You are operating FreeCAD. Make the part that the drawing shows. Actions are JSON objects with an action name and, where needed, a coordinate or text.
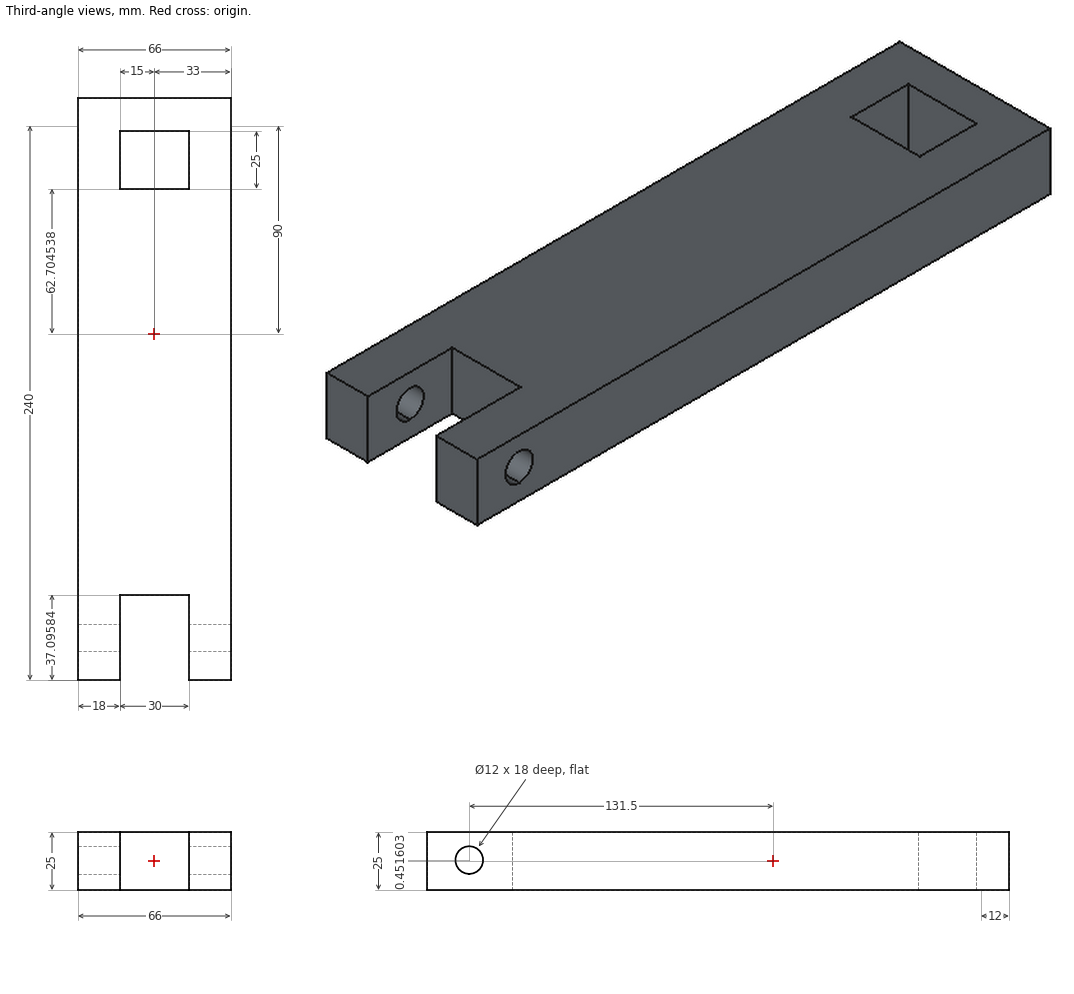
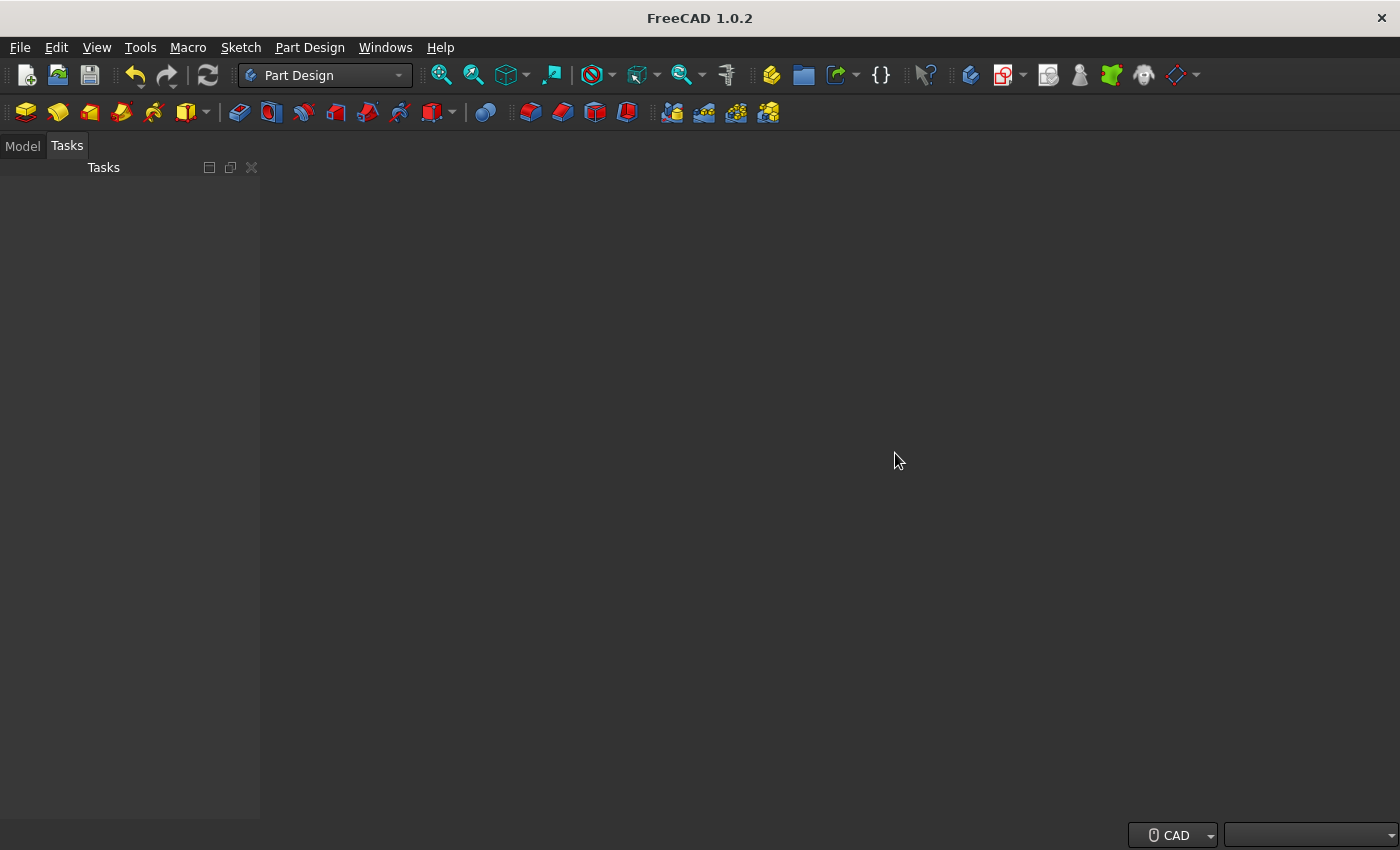
{"action": "left_click", "coordinate": [26, 76]}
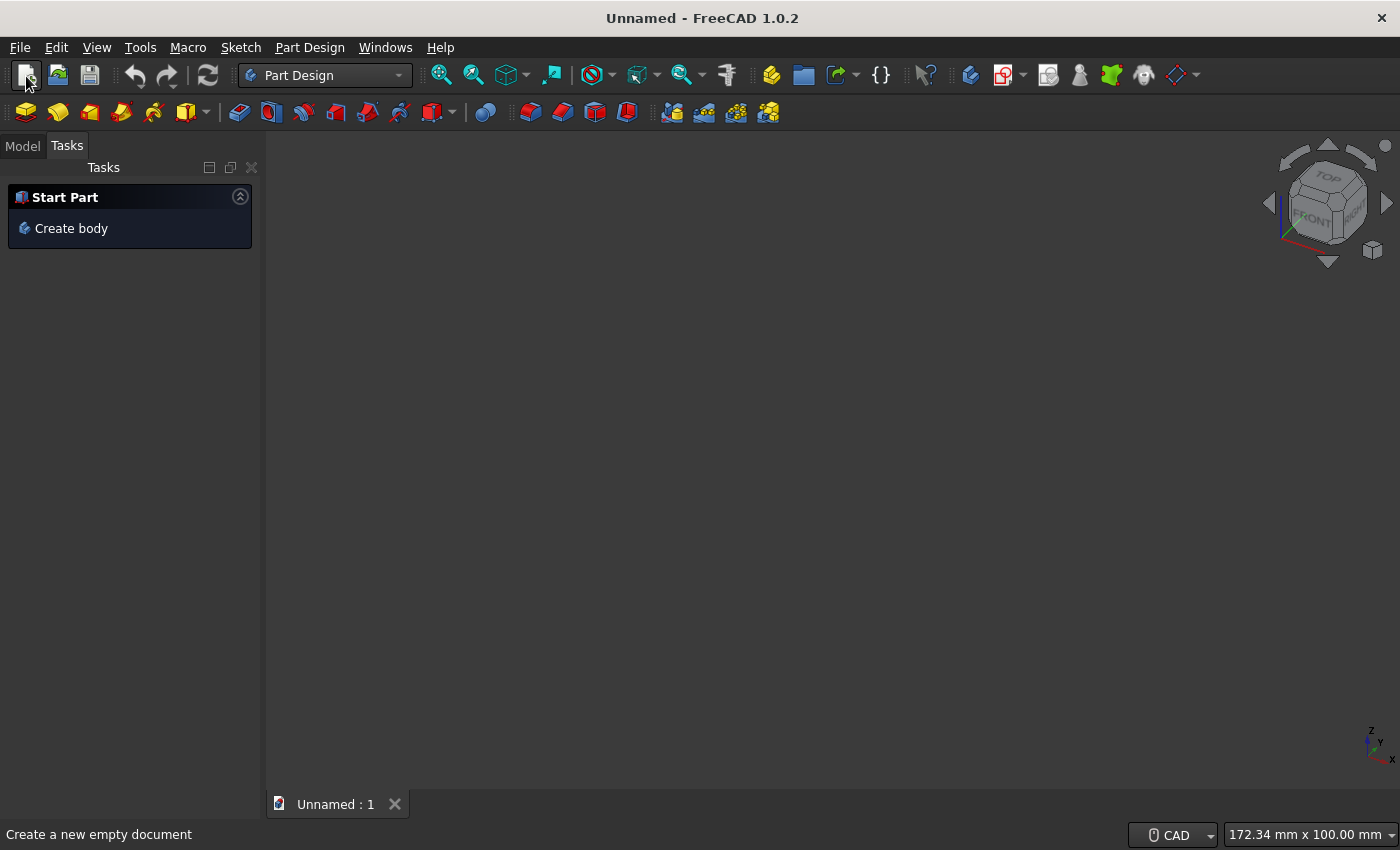
{"action": "left_click", "coordinate": [1004, 76]}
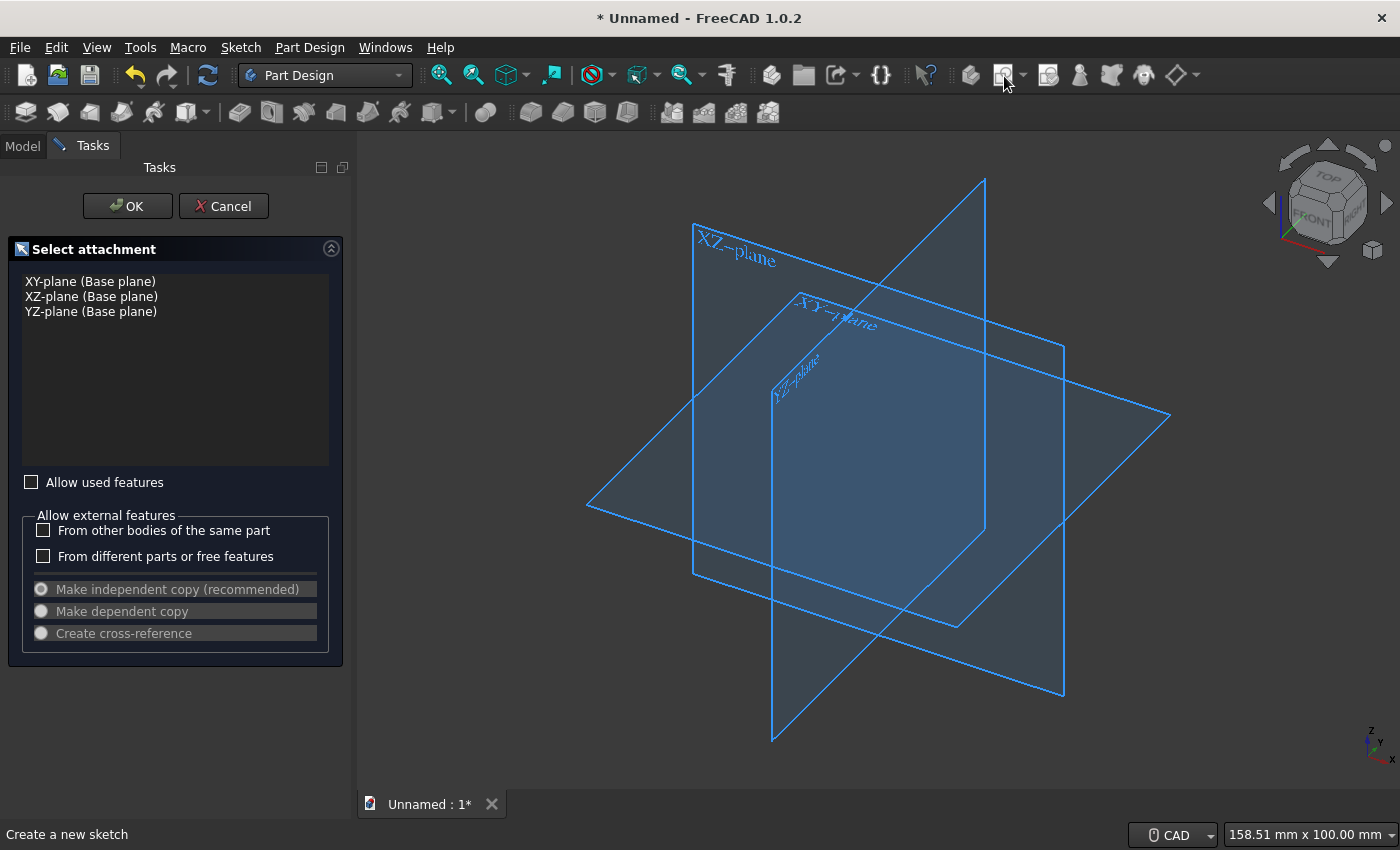
{"action": "left_click", "coordinate": [82, 282]}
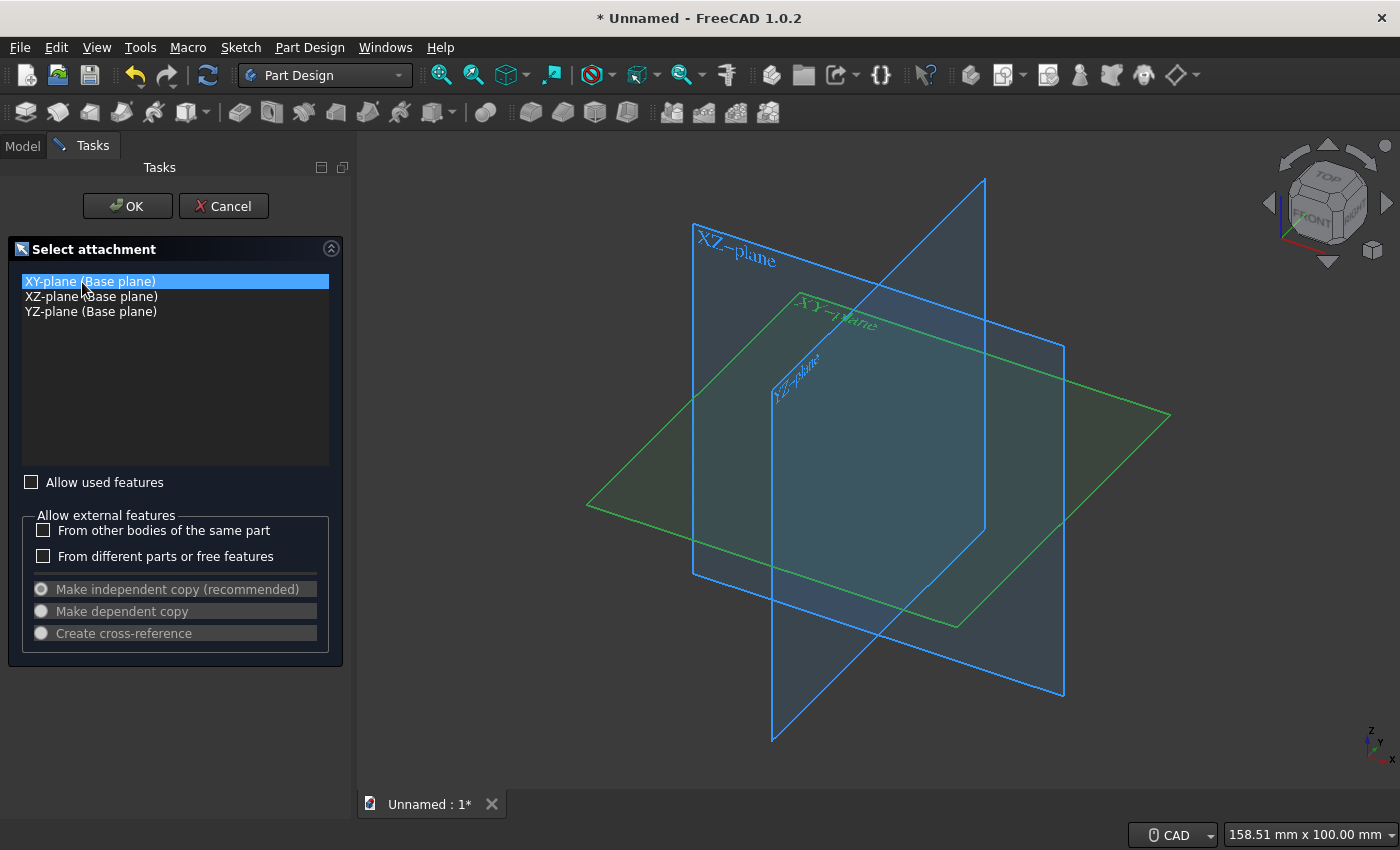
{"action": "left_click", "coordinate": [128, 206]}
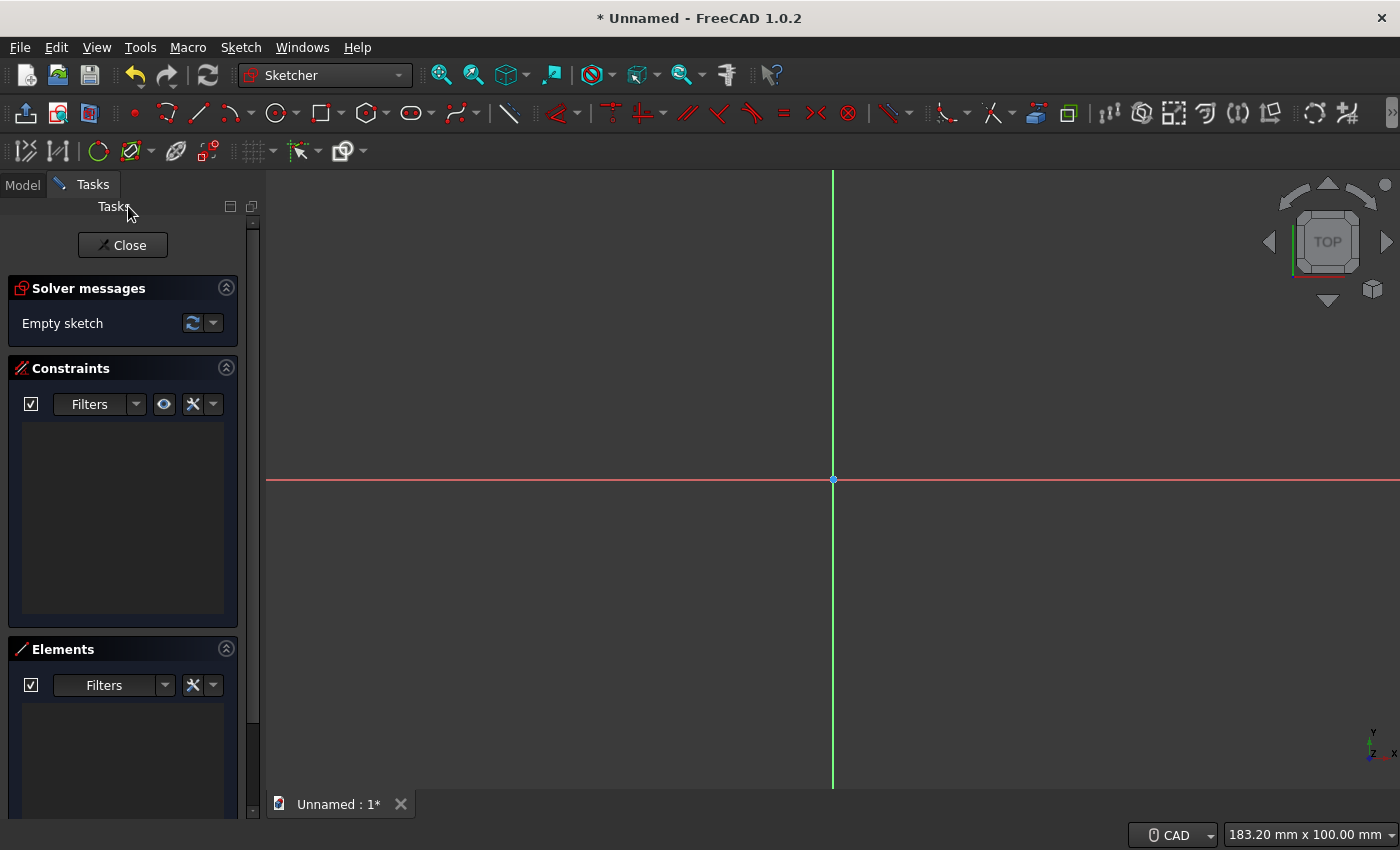
{"action": "scroll", "coordinate": [742, 419], "scroll_direction": "down", "scroll_amount": 7}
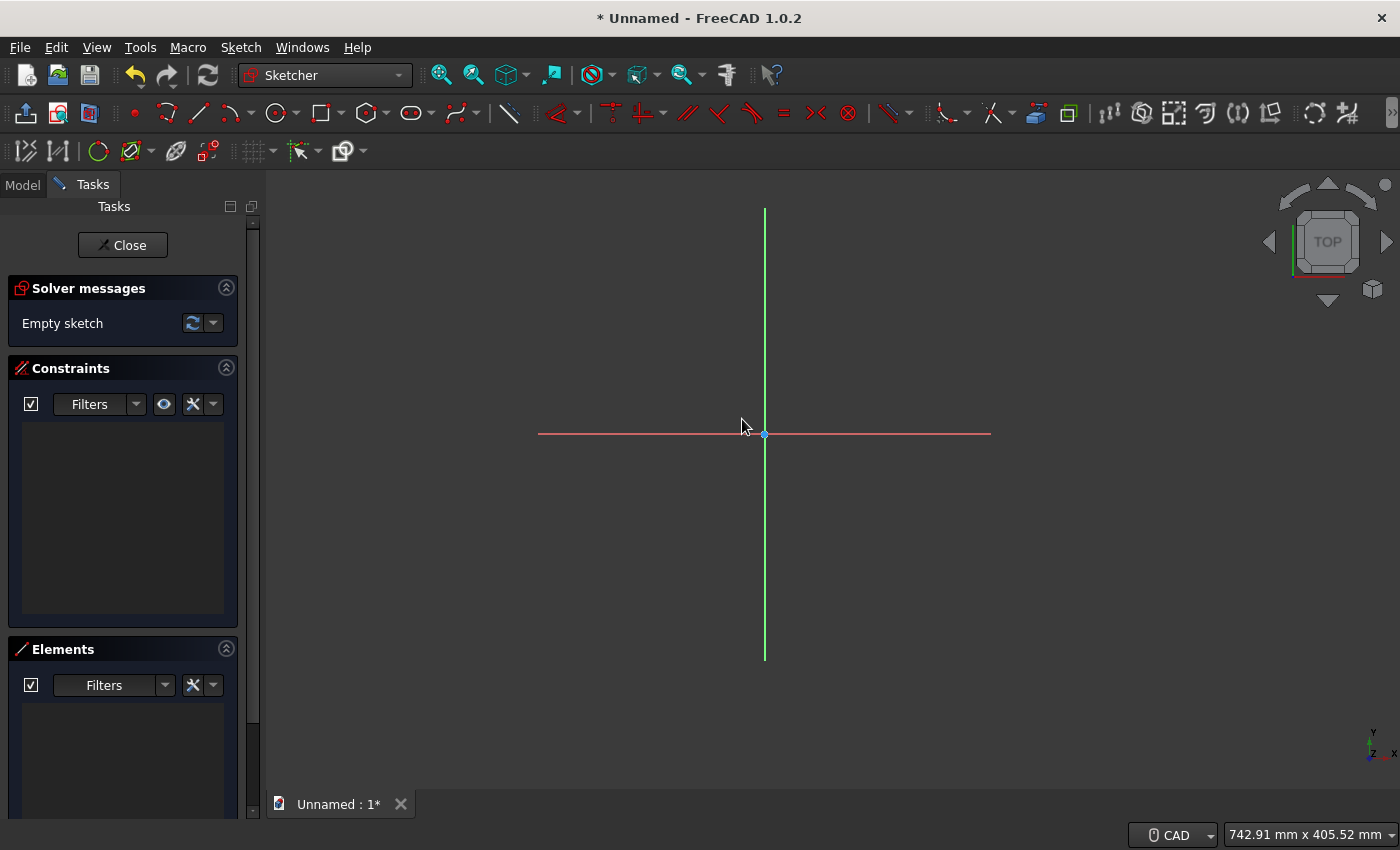
{"action": "left_click", "coordinate": [168, 114]}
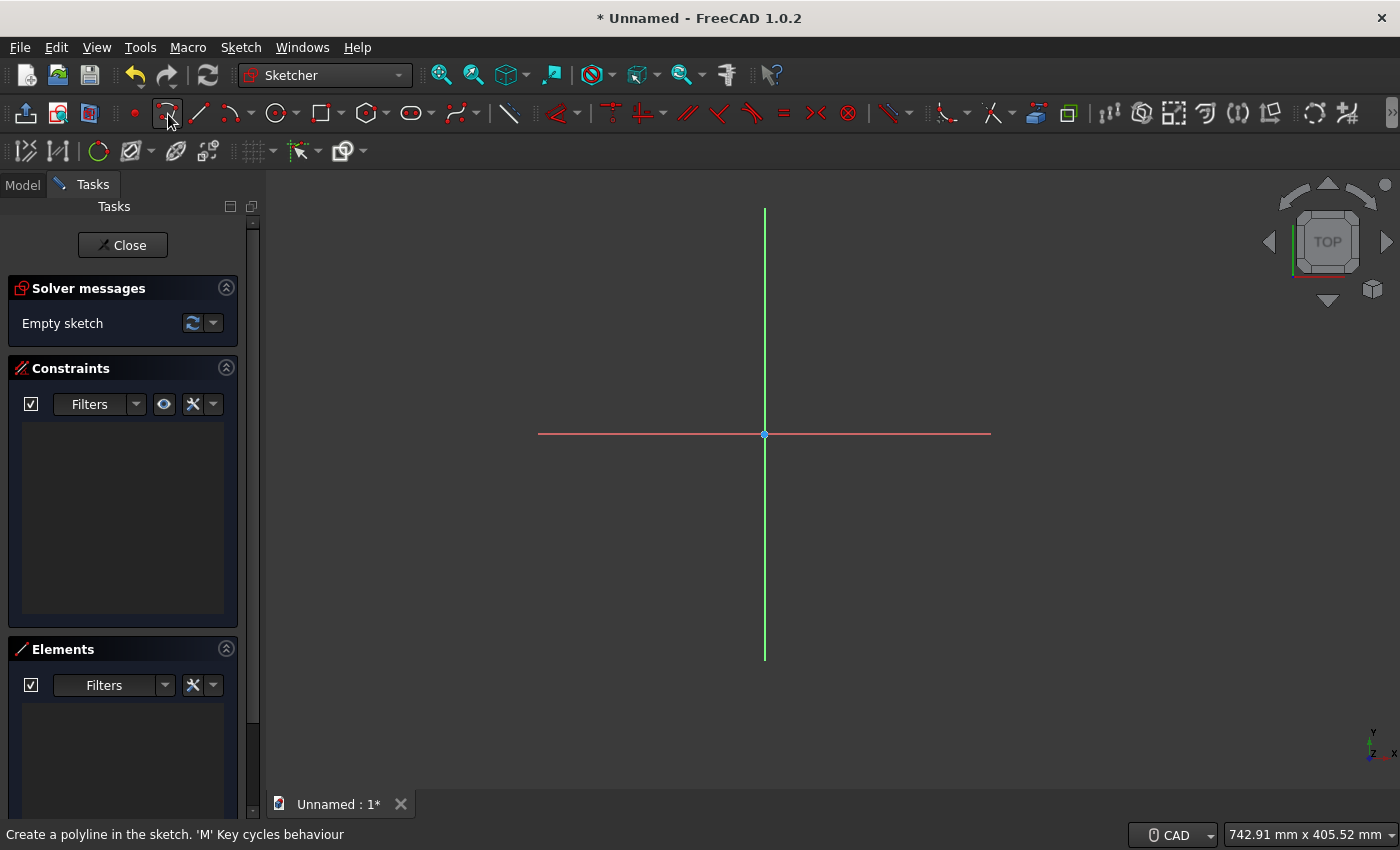
{"action": "left_click", "coordinate": [815, 297]}
{"action": "left_click", "coordinate": [714, 297]}
{"action": "left_click", "coordinate": [714, 663]}
{"action": "left_click", "coordinate": [742, 663]}
{"action": "left_click", "coordinate": [742, 607]}
{"action": "left_click", "coordinate": [788, 607]}
{"action": "left_click", "coordinate": [788, 663]}
{"action": "left_click", "coordinate": [815, 663]}
{"action": "left_click", "coordinate": [815, 298]}
{"action": "key", "text": "Escape"}
{"action": "key", "text": "Escape"}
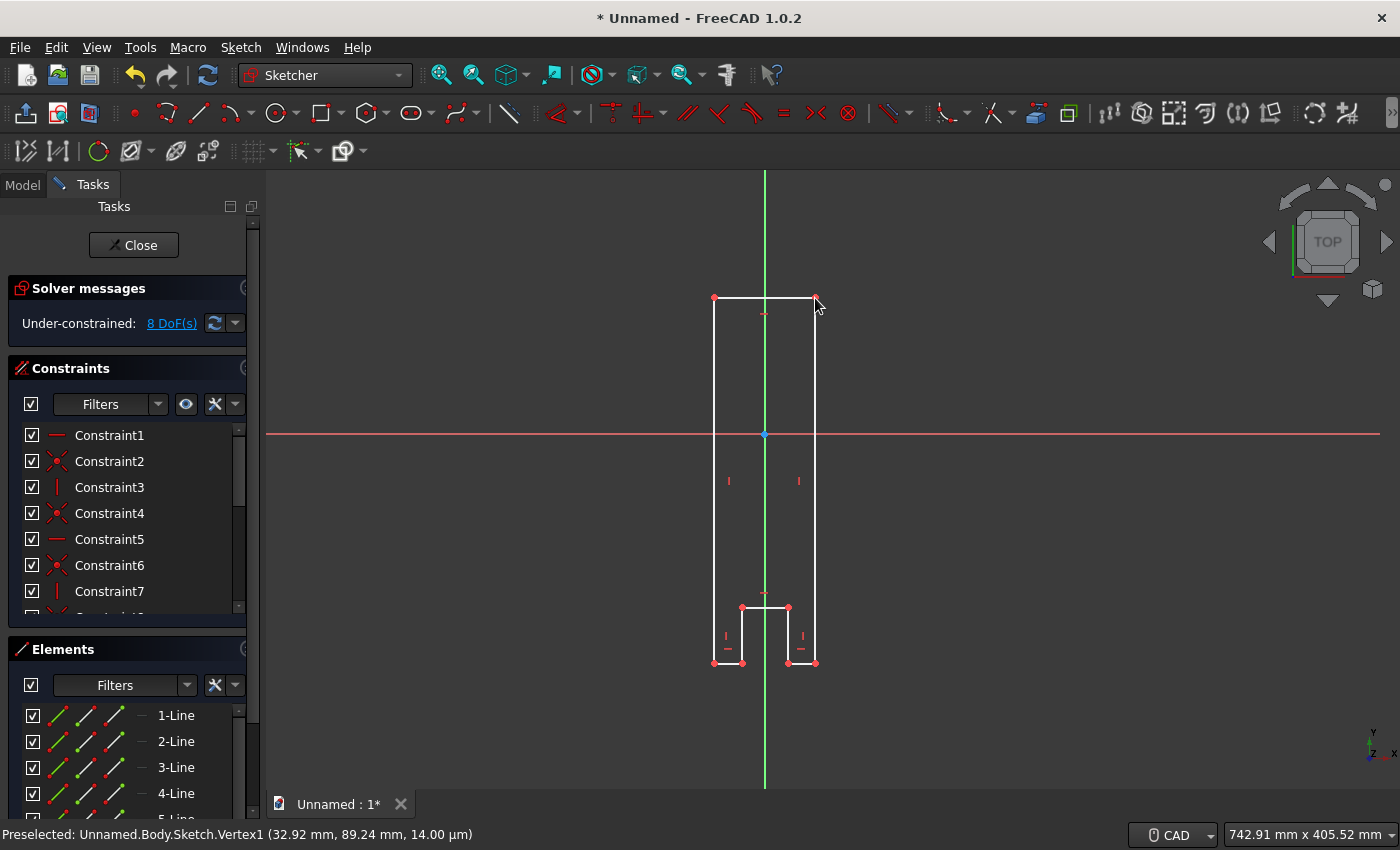
{"action": "left_click", "coordinate": [556, 114]}